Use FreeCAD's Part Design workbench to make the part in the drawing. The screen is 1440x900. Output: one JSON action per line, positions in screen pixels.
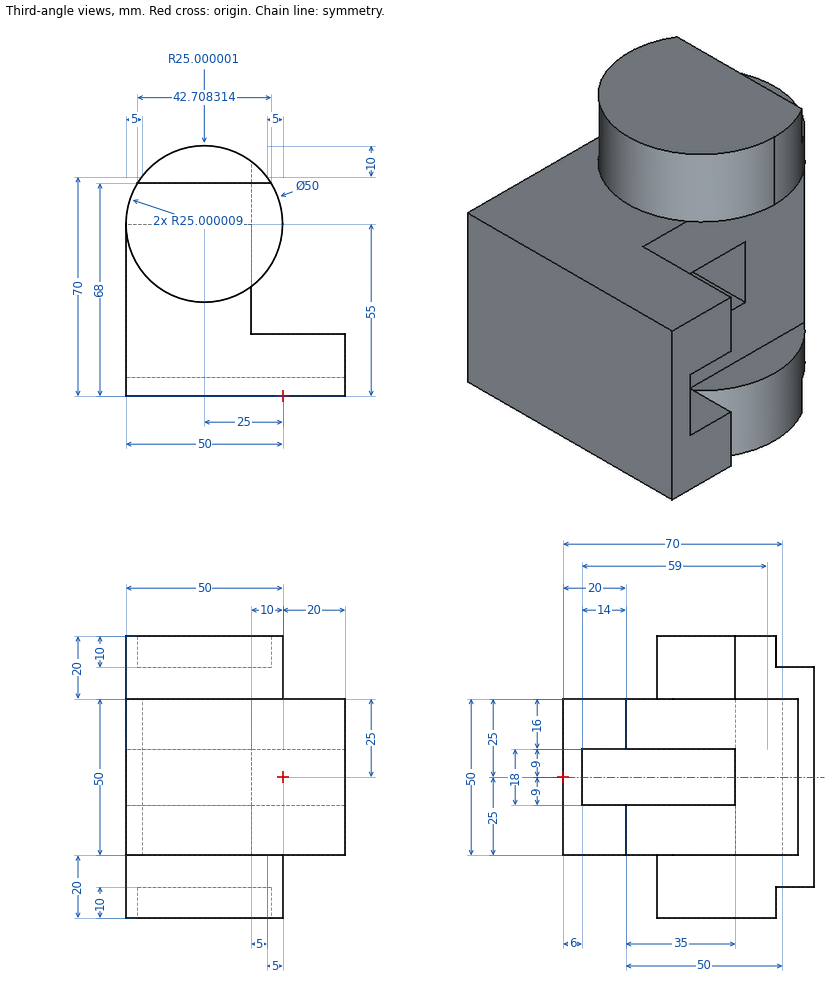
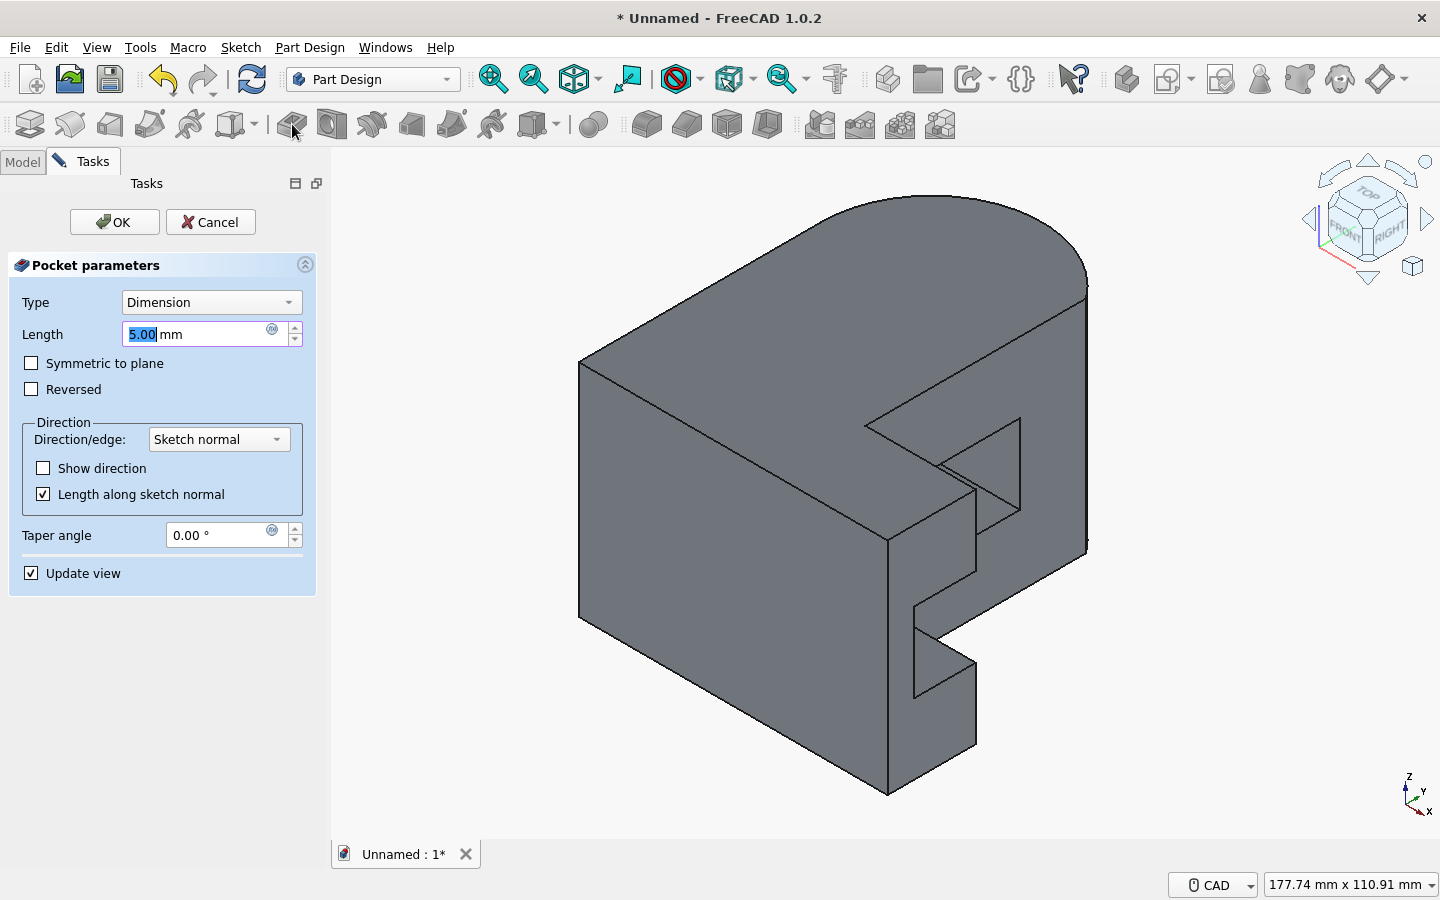
{"action": "type", "text": "10"}
{"action": "key", "text": "Tab"}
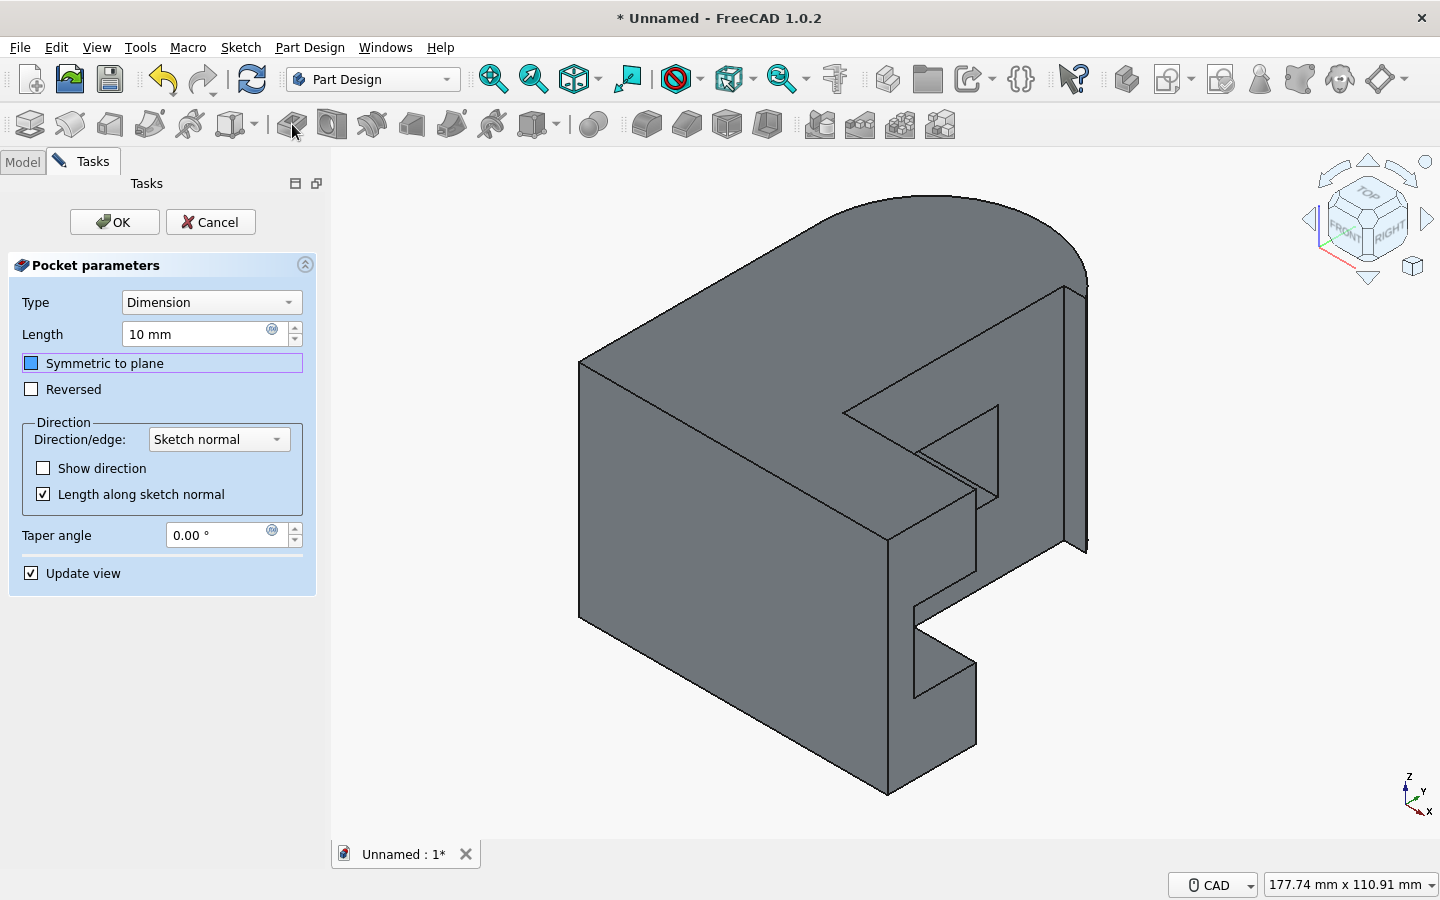
{"action": "left_click", "coordinate": [115, 222]}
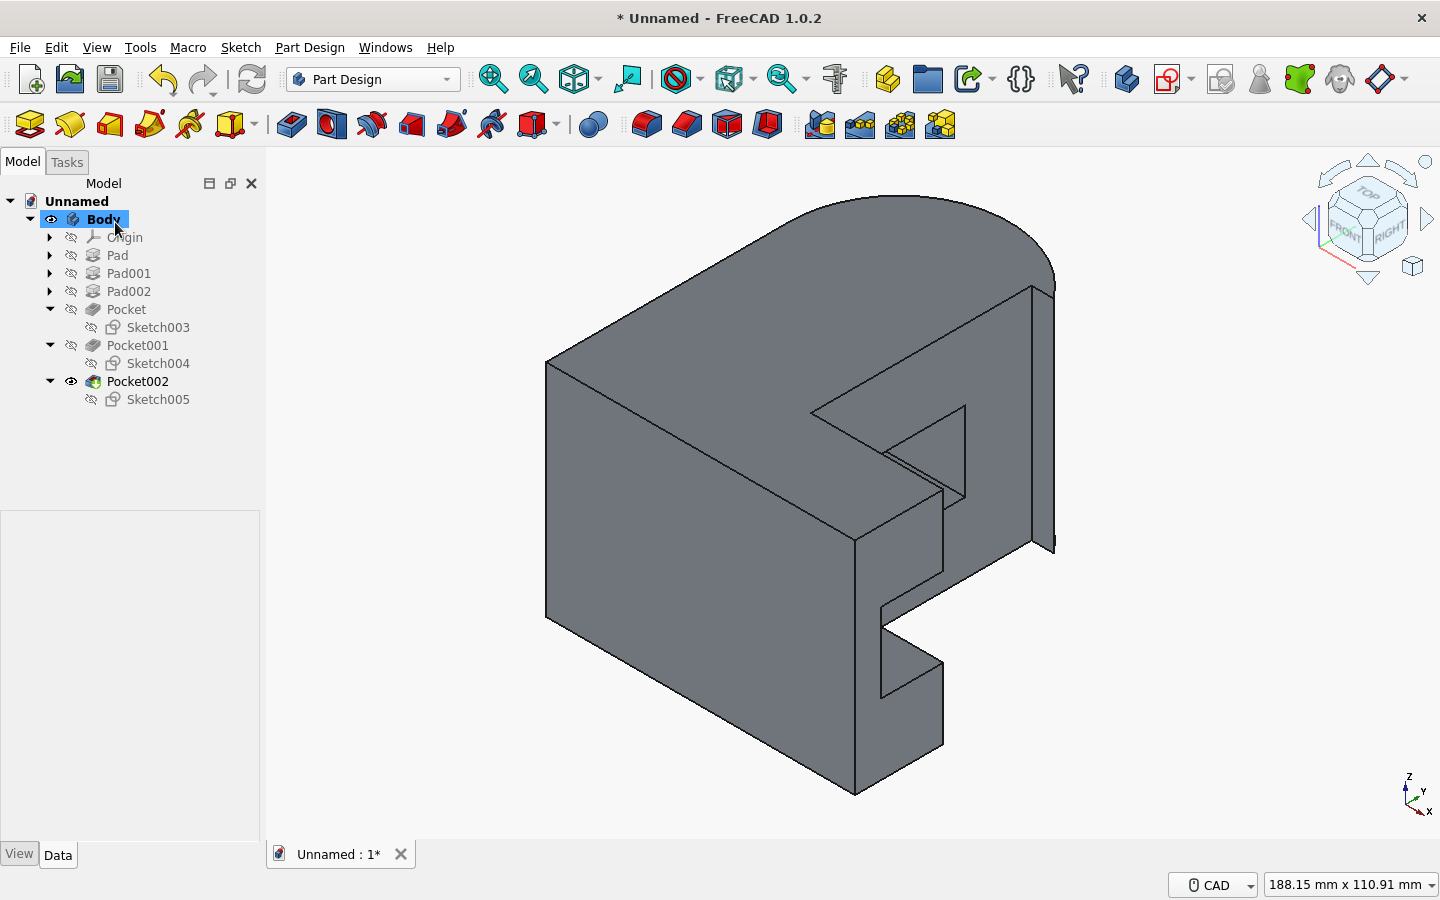
{"action": "left_click", "coordinate": [50, 237]}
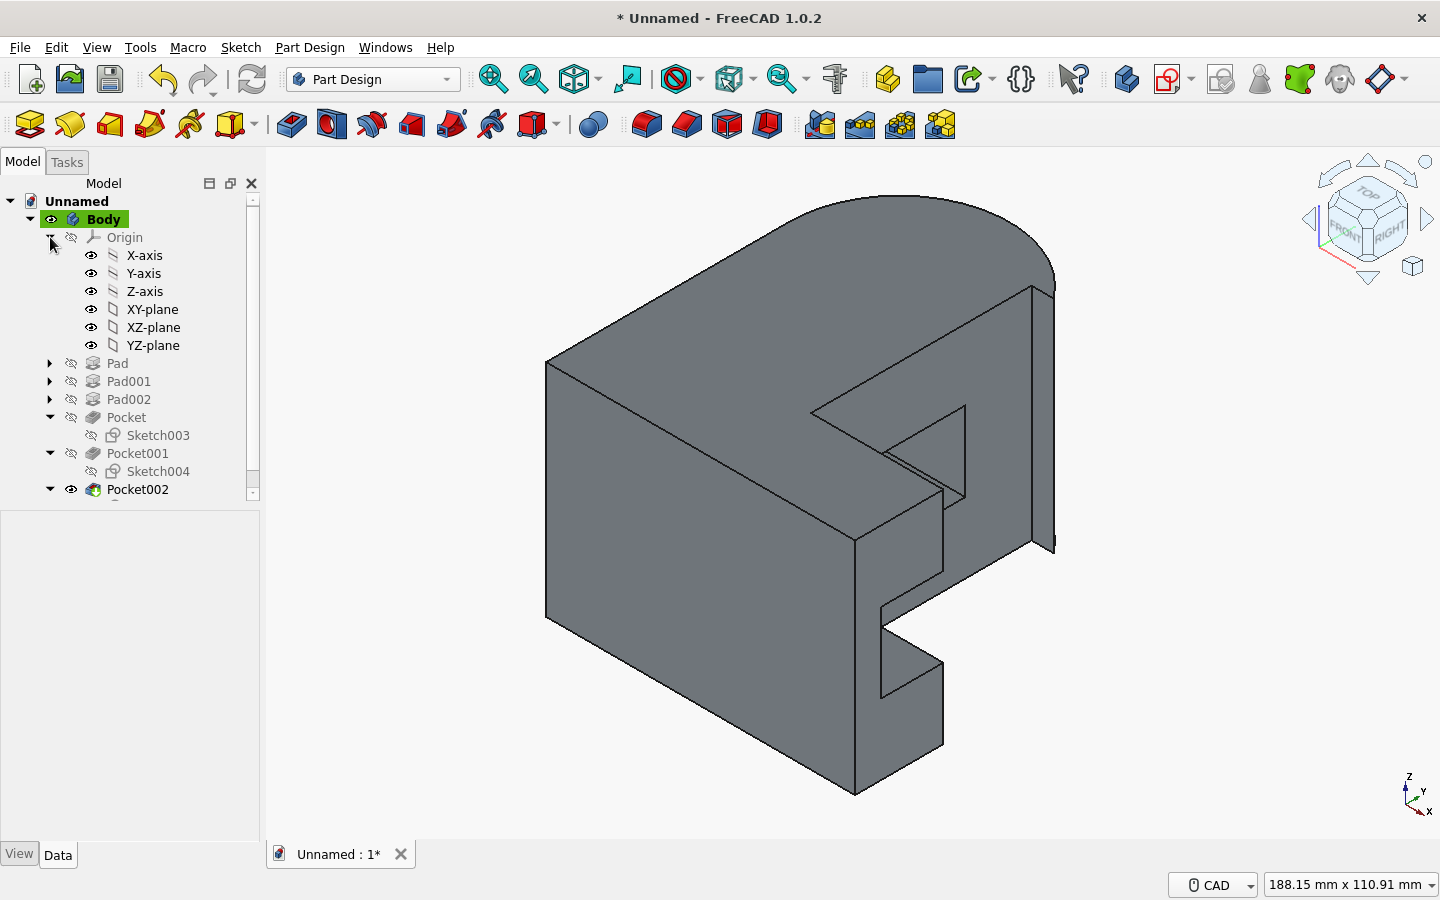
{"action": "left_click", "coordinate": [136, 327]}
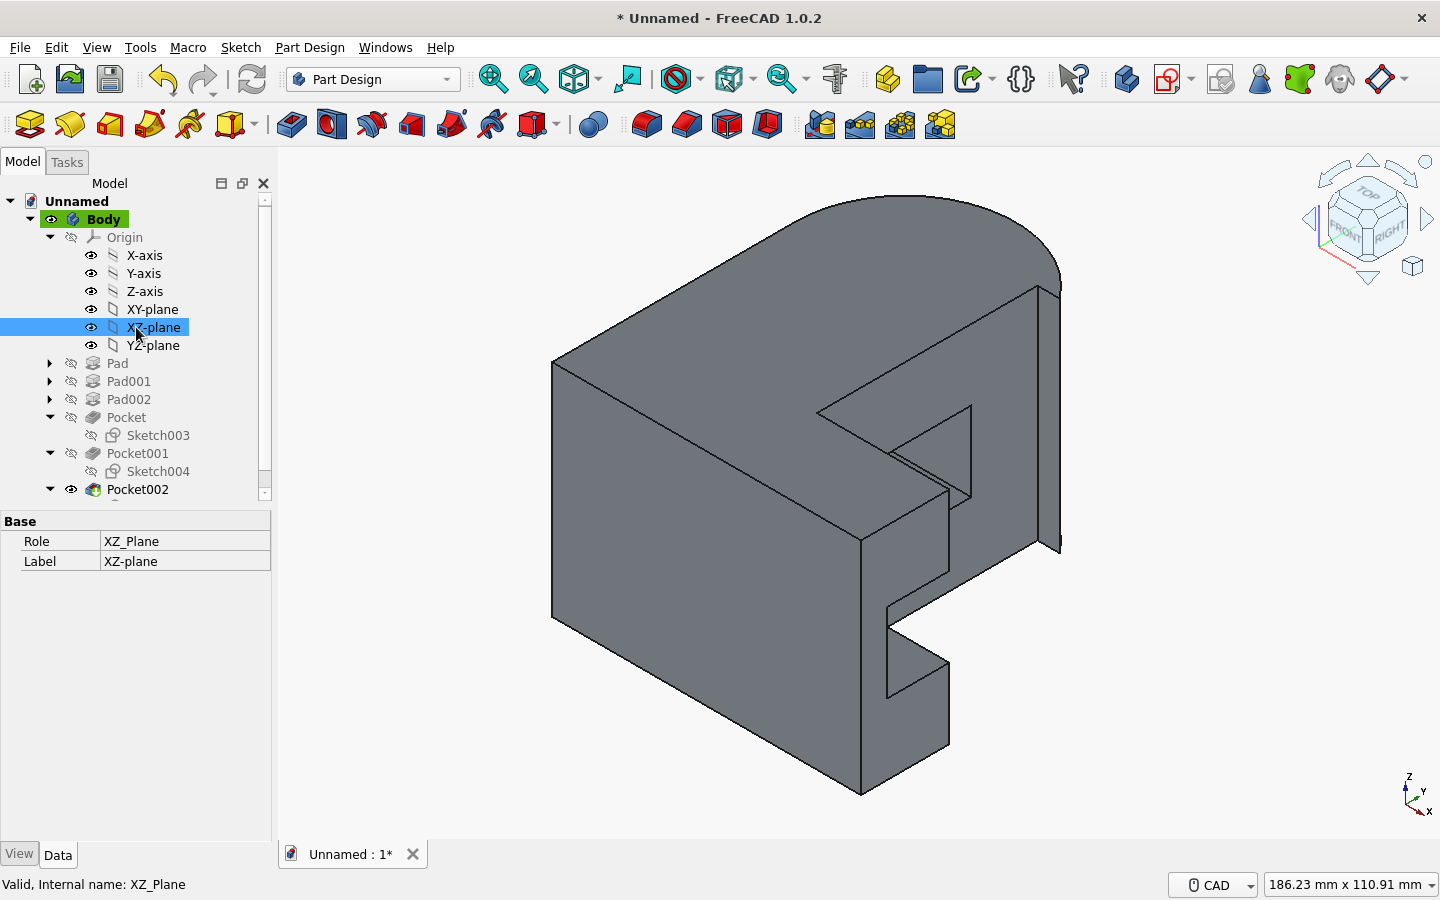
{"action": "left_click", "coordinate": [1380, 80]}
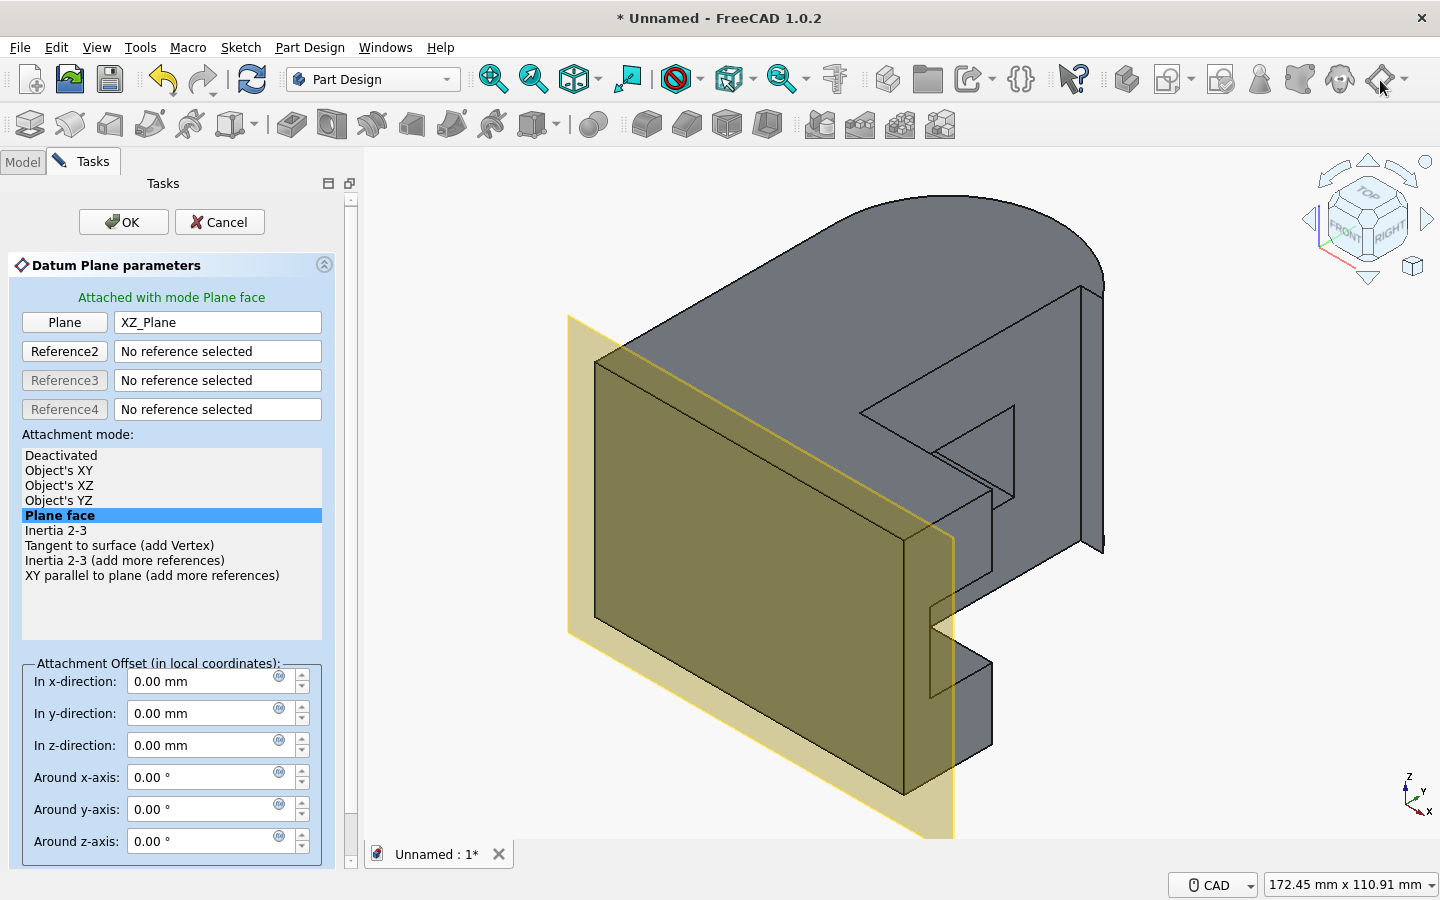
{"action": "triple_click", "coordinate": [210, 745]}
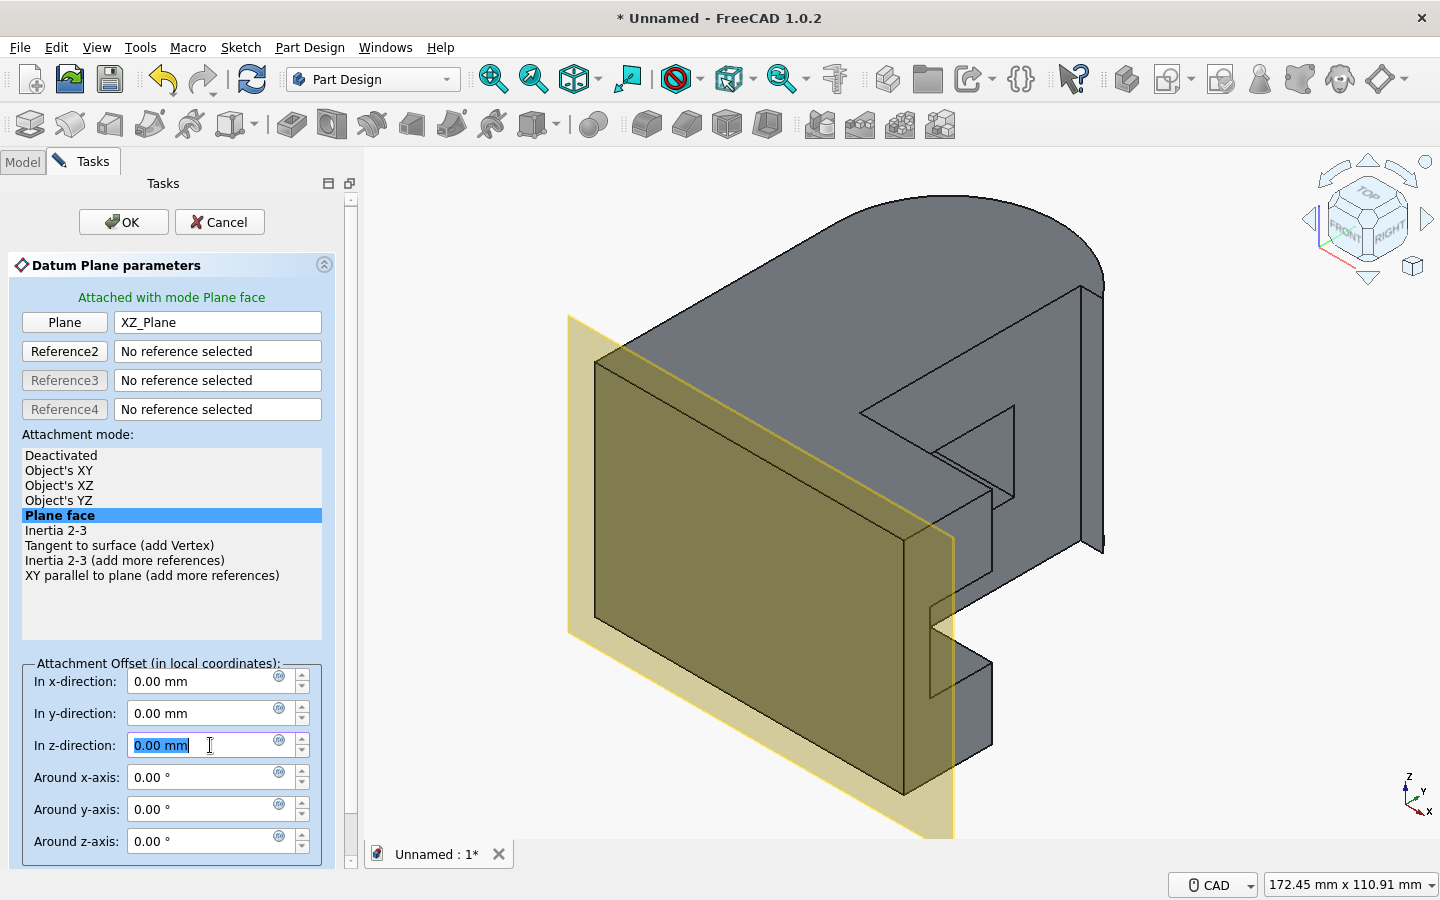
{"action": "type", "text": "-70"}
{"action": "key", "text": "Tab"}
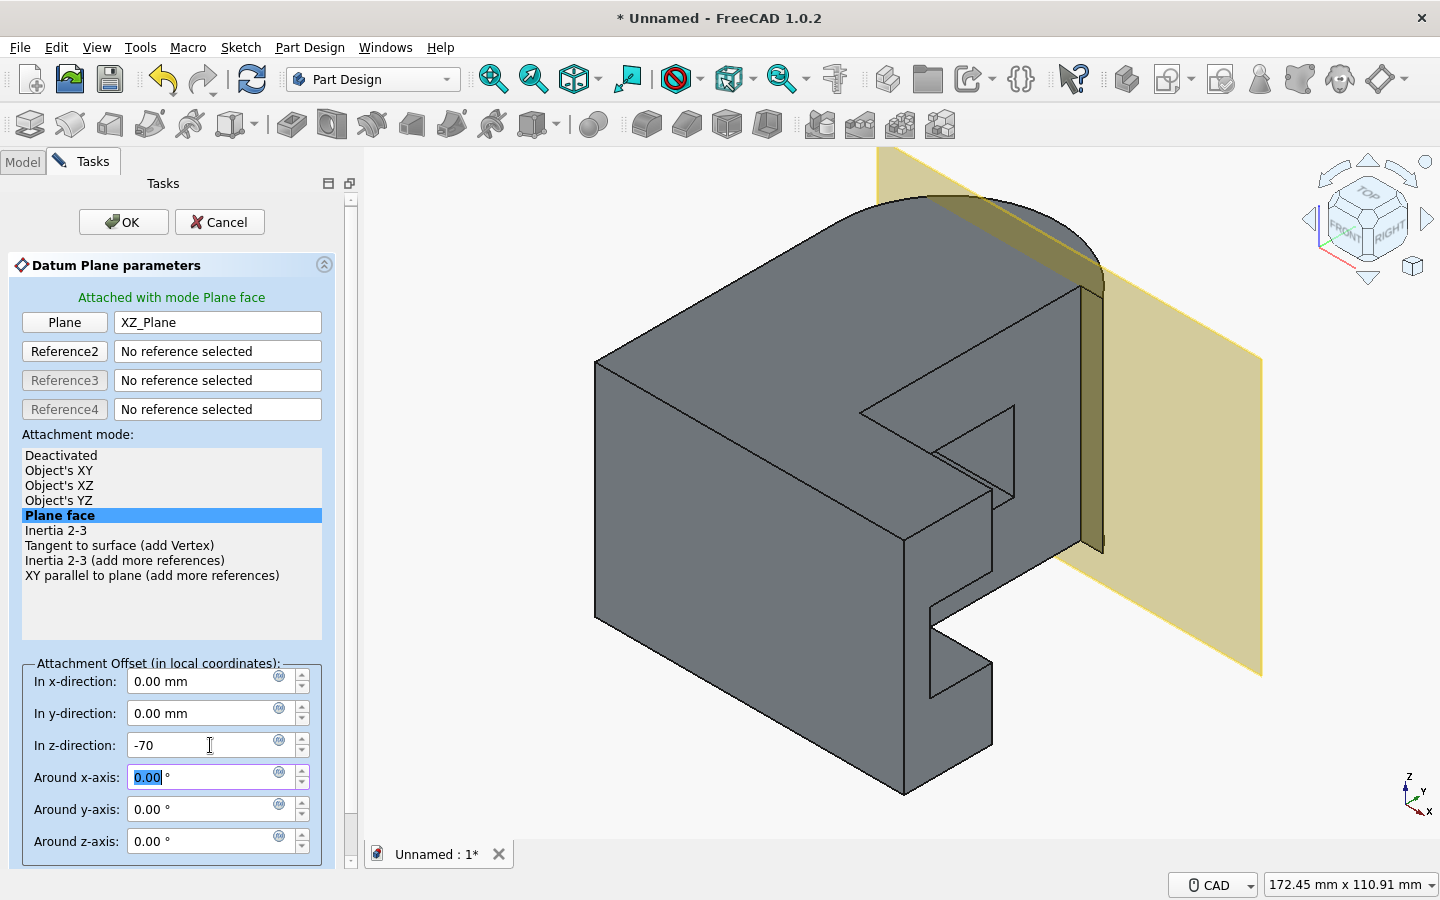
{"action": "left_click", "coordinate": [124, 222]}